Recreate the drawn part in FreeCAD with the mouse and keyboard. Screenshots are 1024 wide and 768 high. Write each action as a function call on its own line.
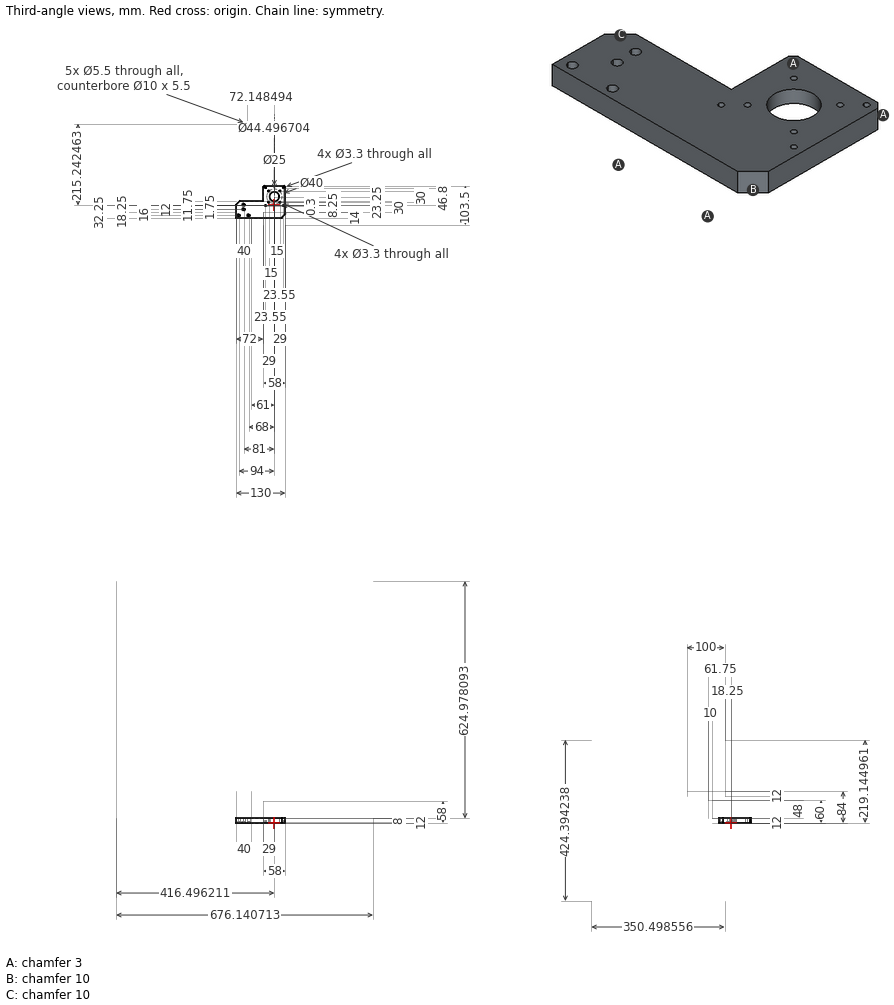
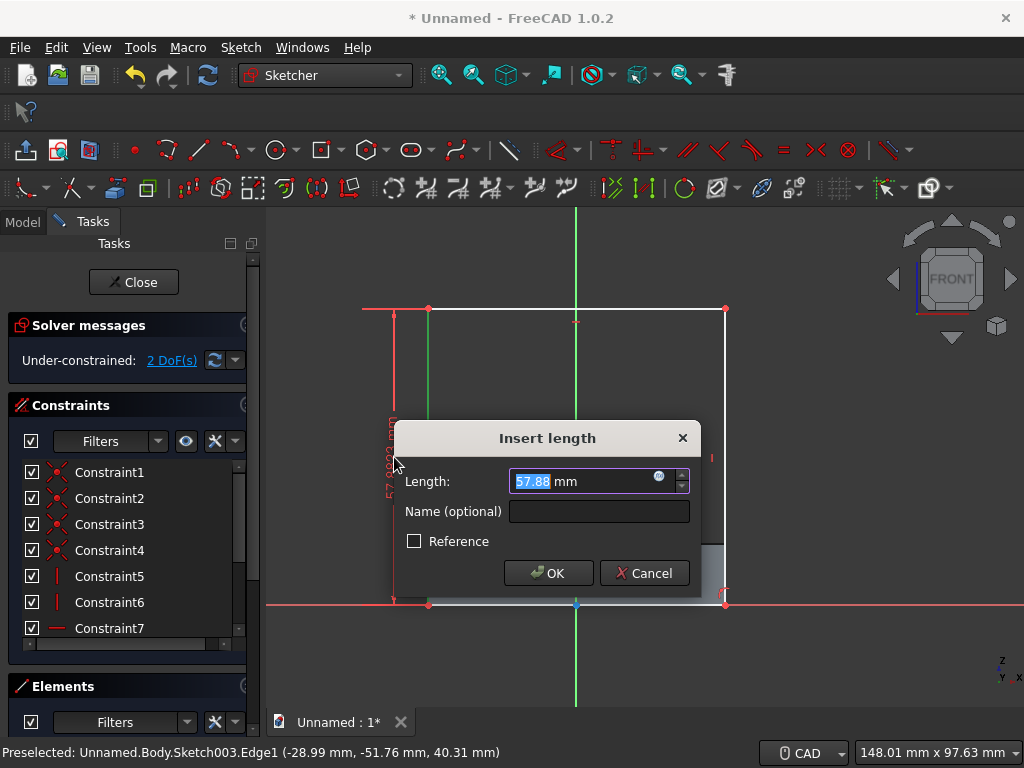
text(58)
key(Return)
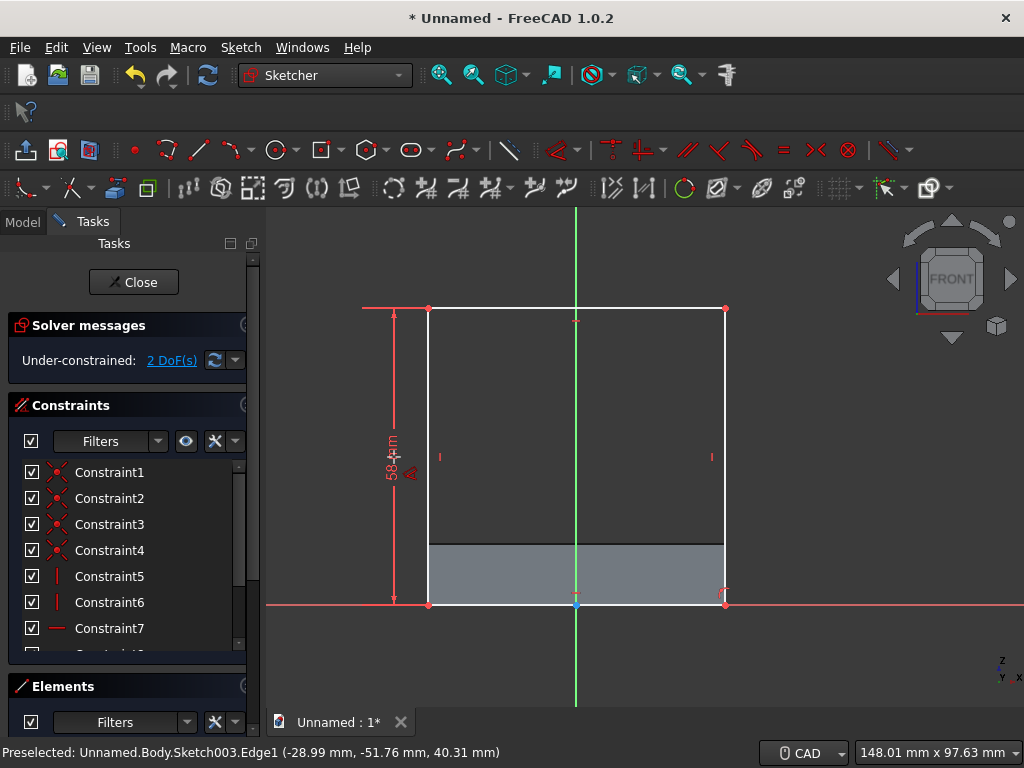
click(517, 605)
click(508, 639)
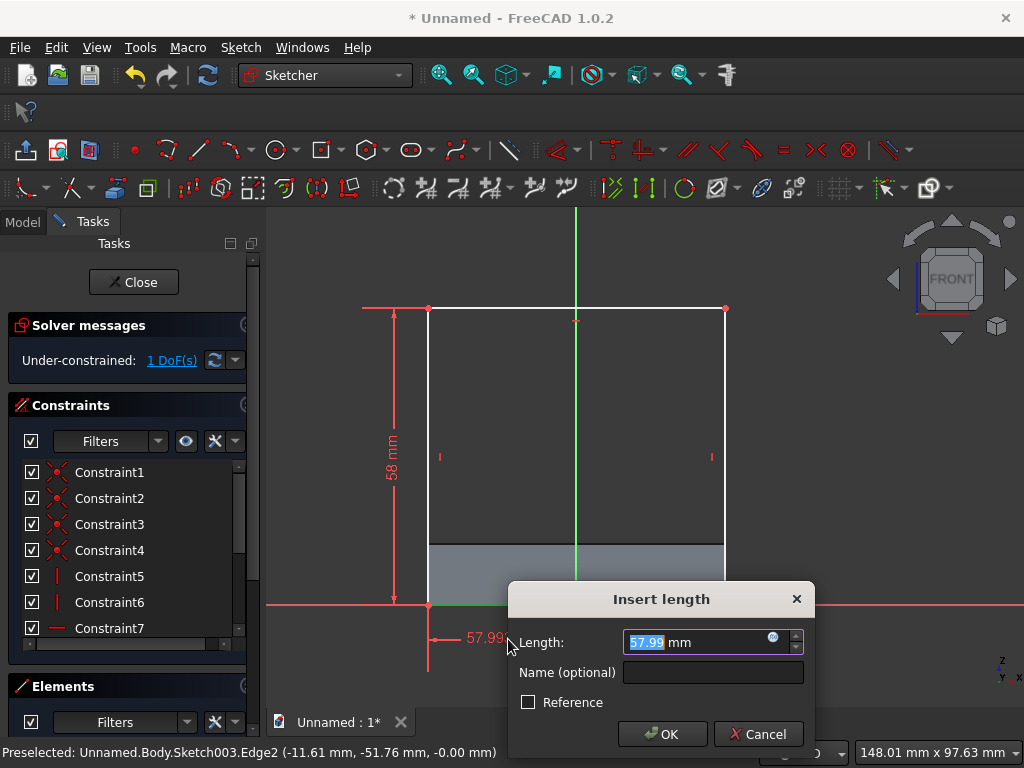
text(58)
key(Return)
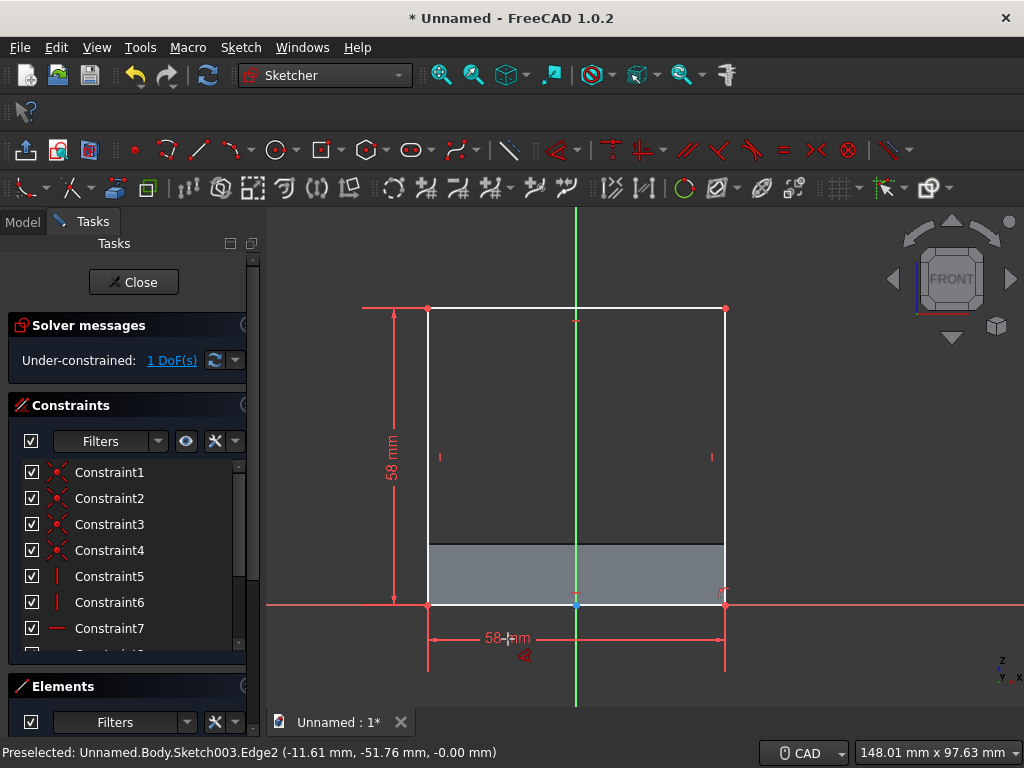
click(428, 308)
click(502, 274)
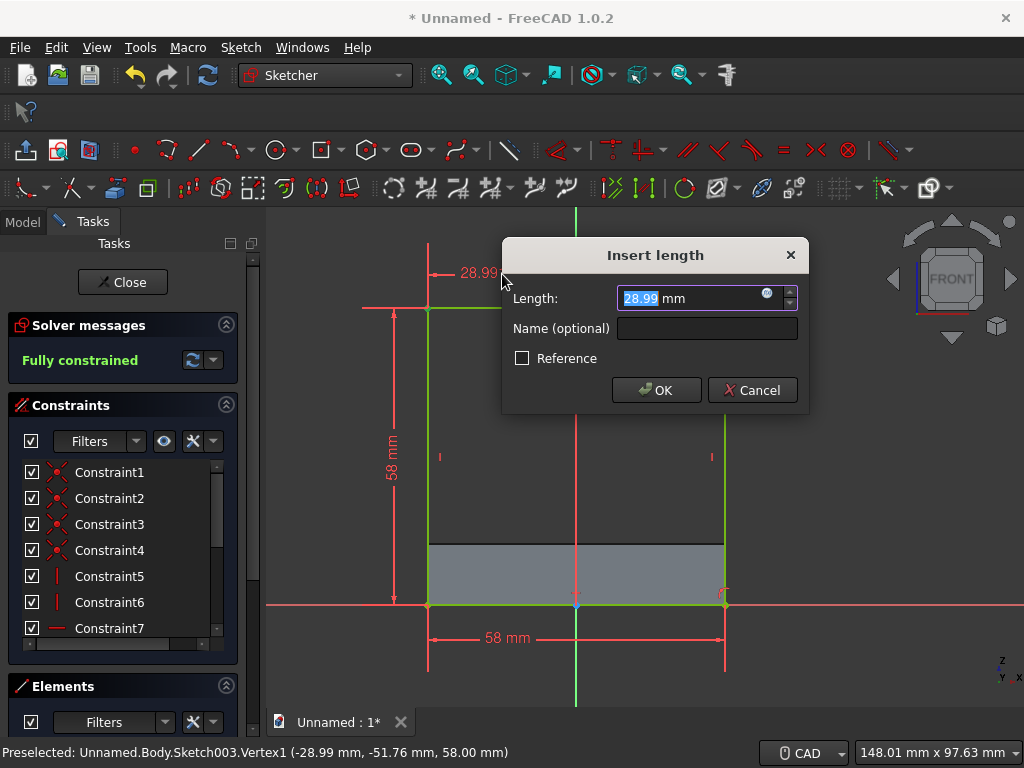
text(29)
key(Return)
key(Escape)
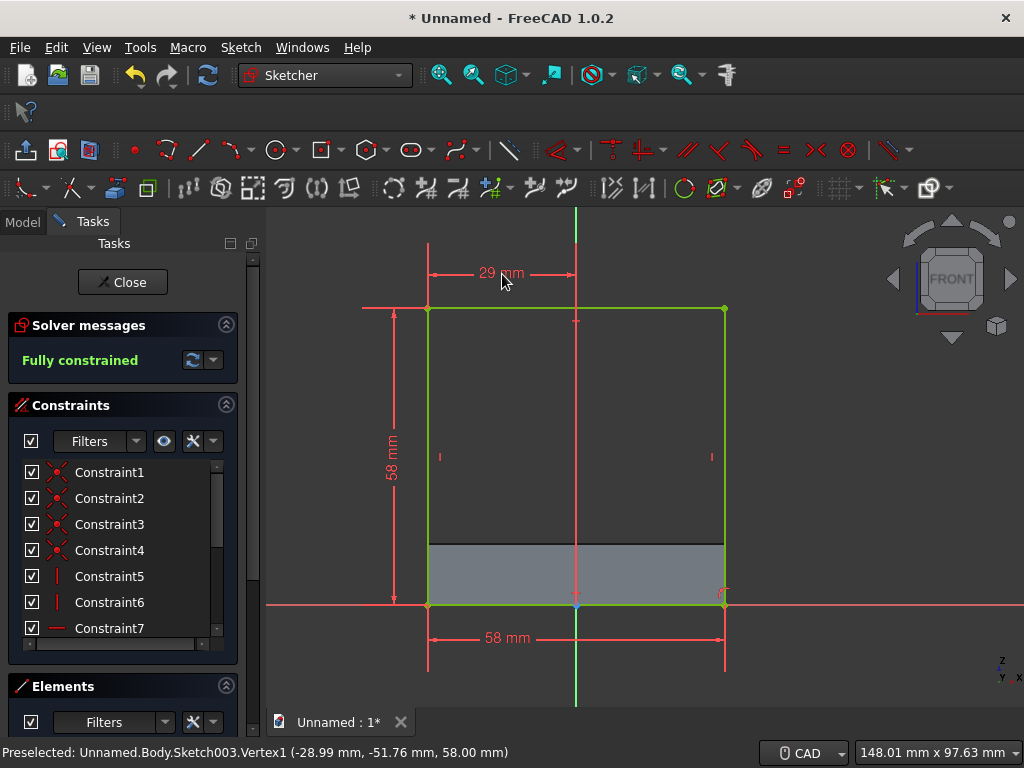
click(123, 282)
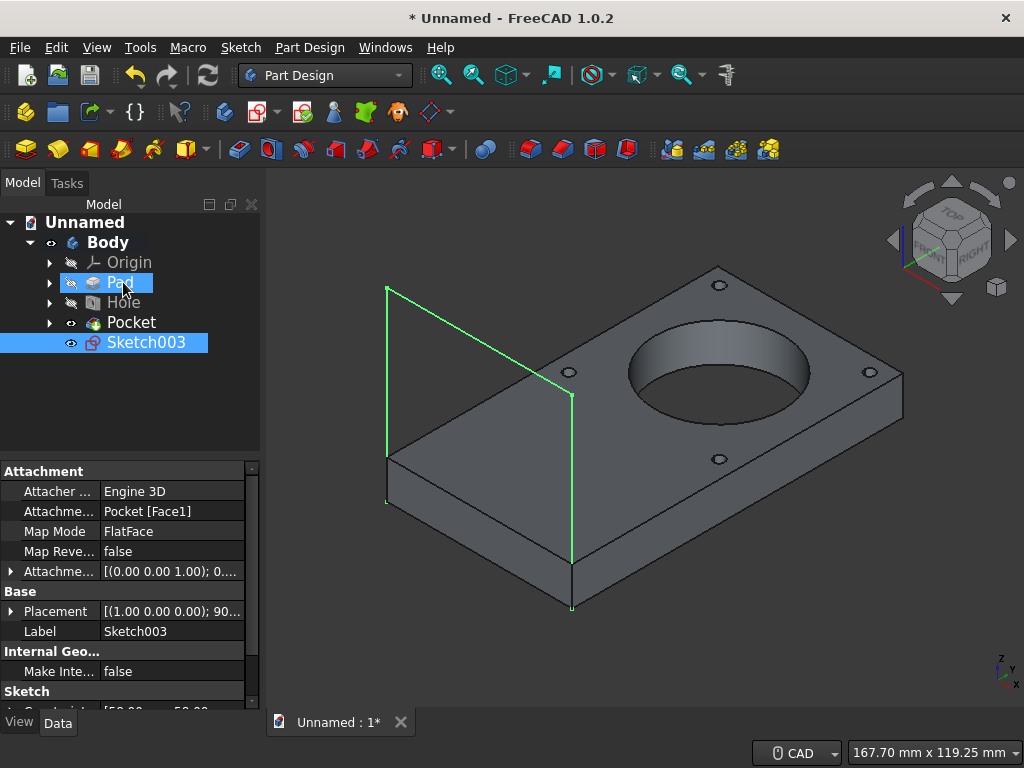
click(26, 150)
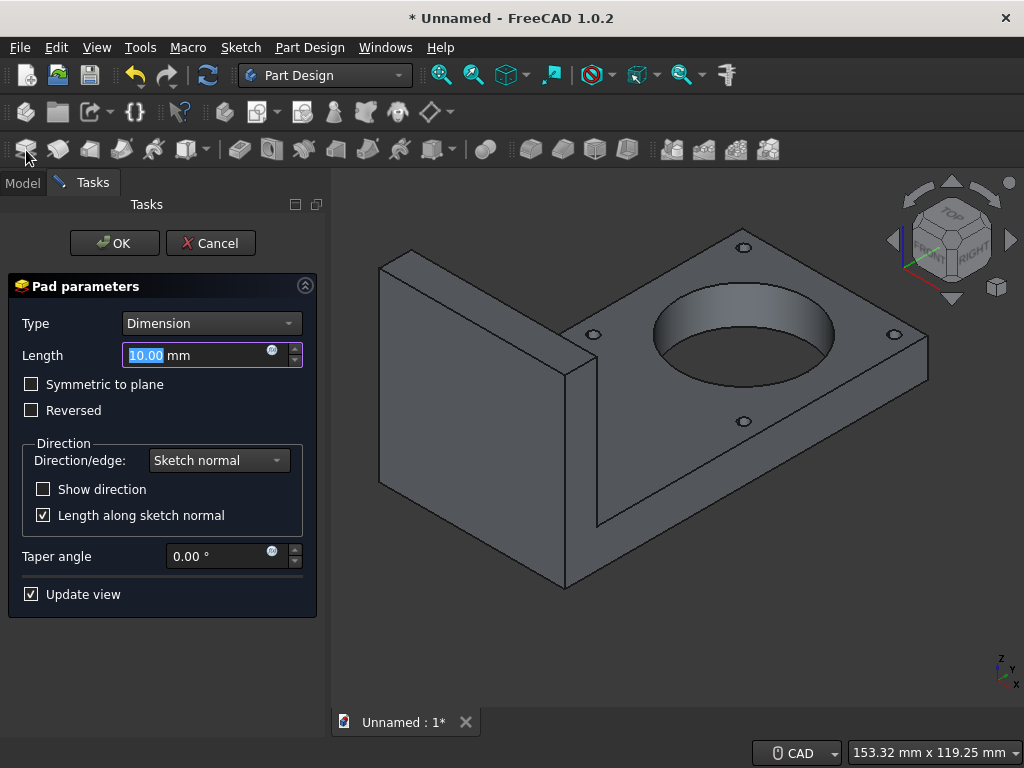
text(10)
key(Tab)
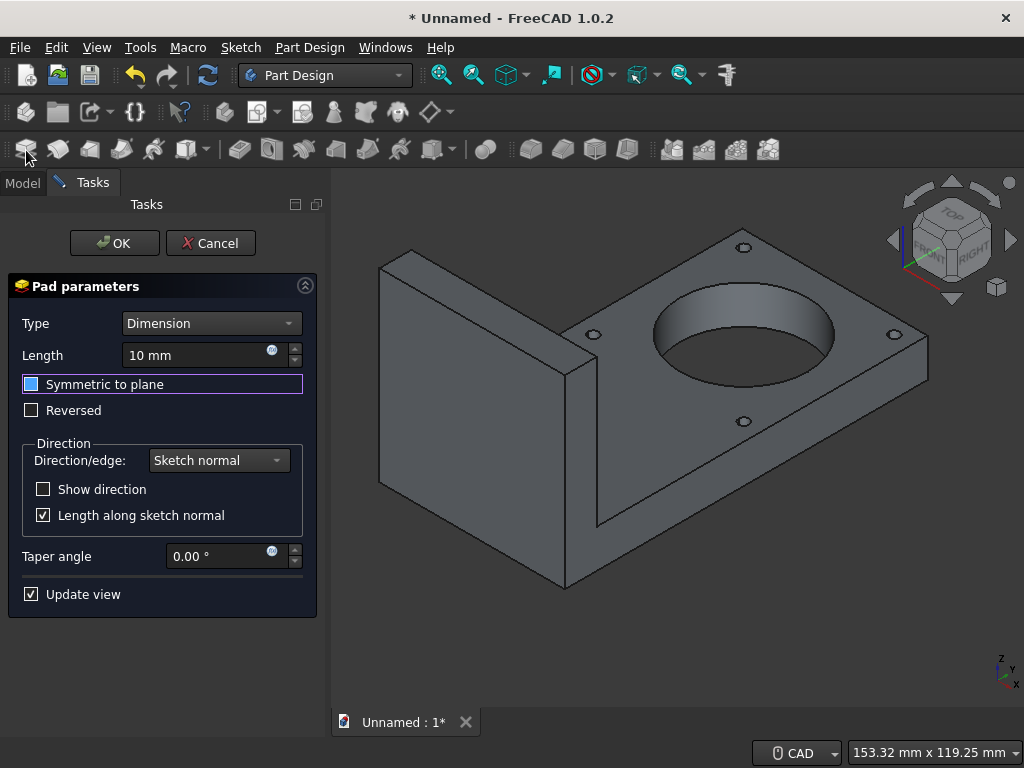
click(115, 243)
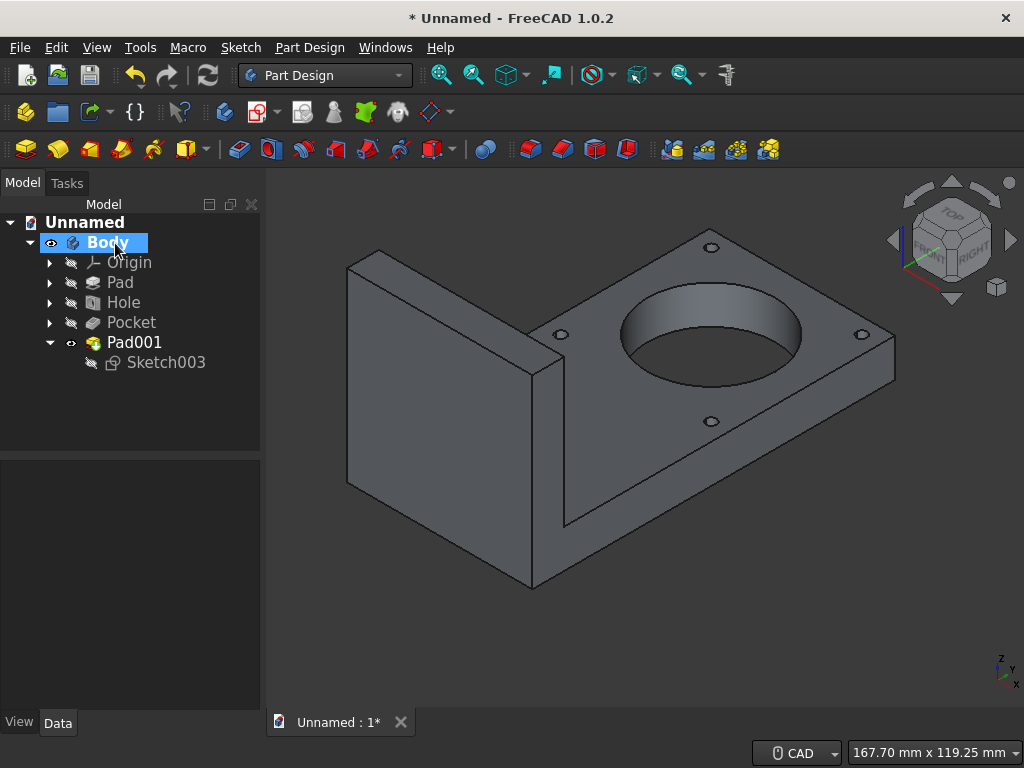
click(442, 76)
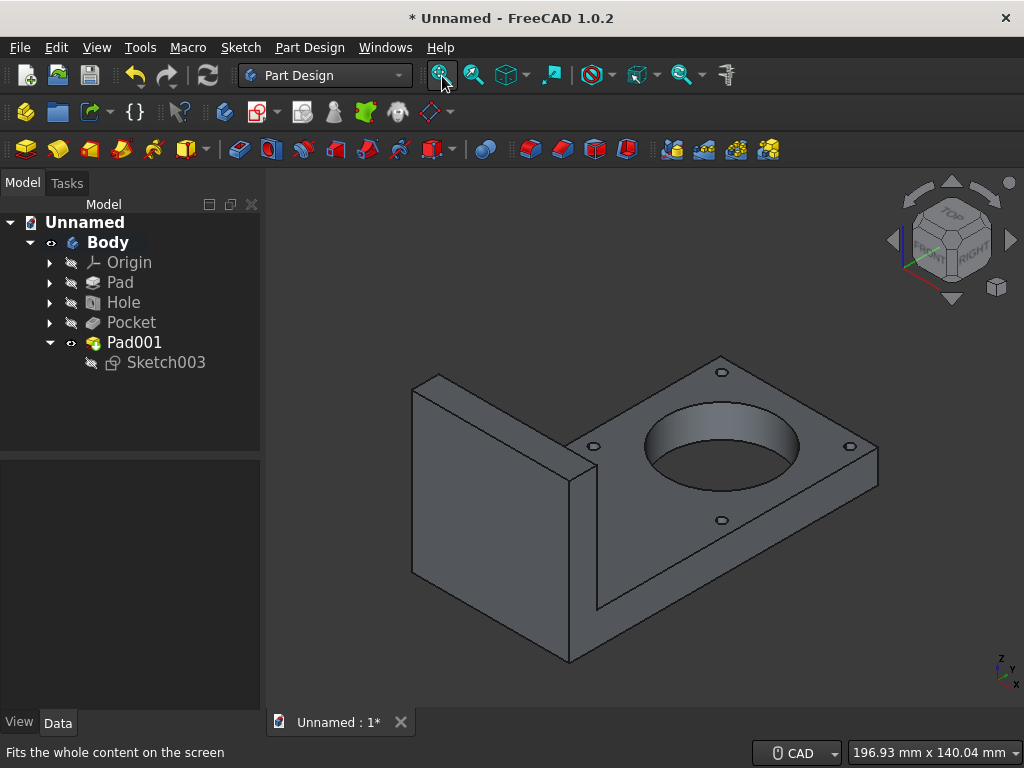
click(856, 484)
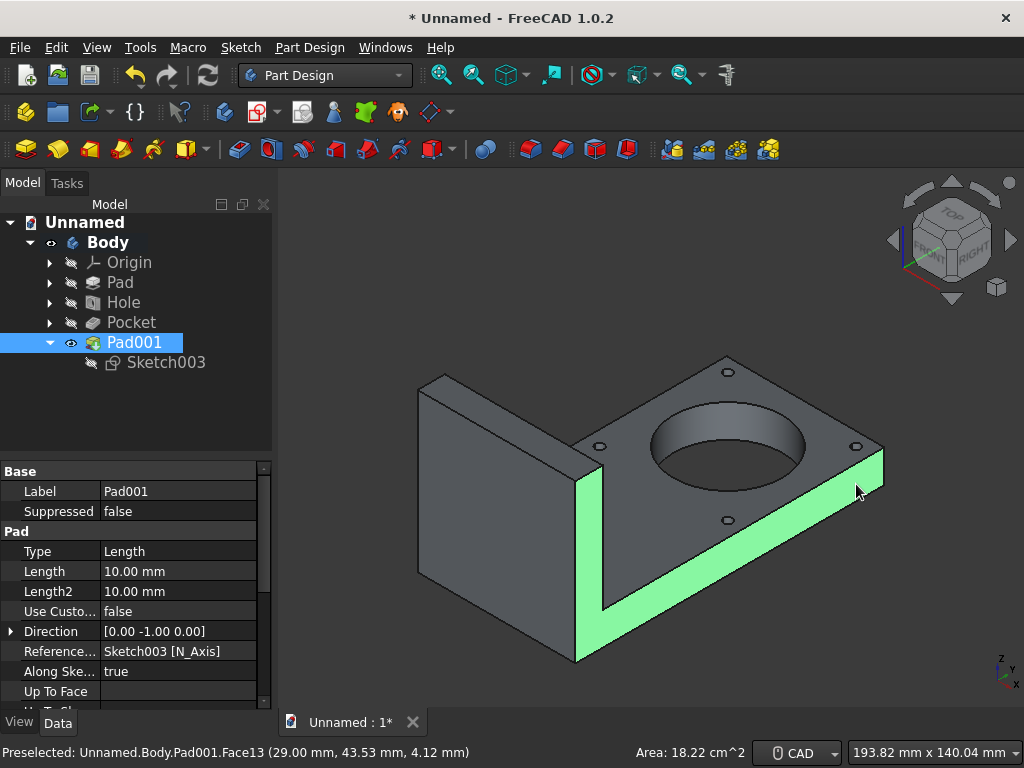
click(258, 112)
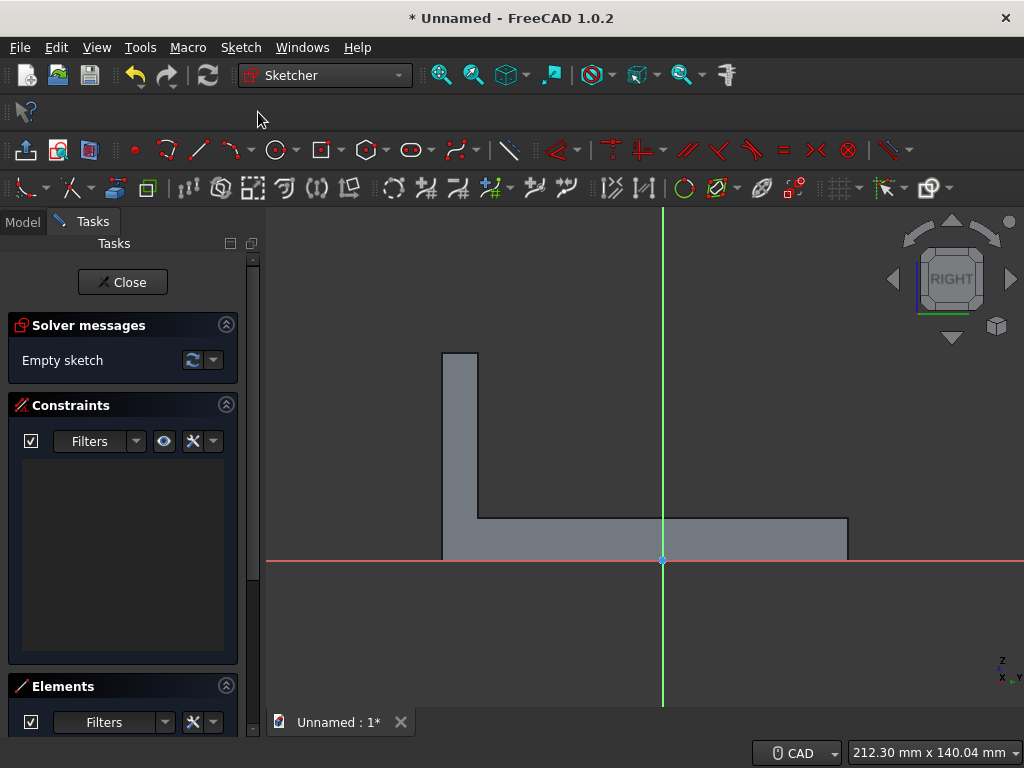
scroll(504, 446, up, 2)